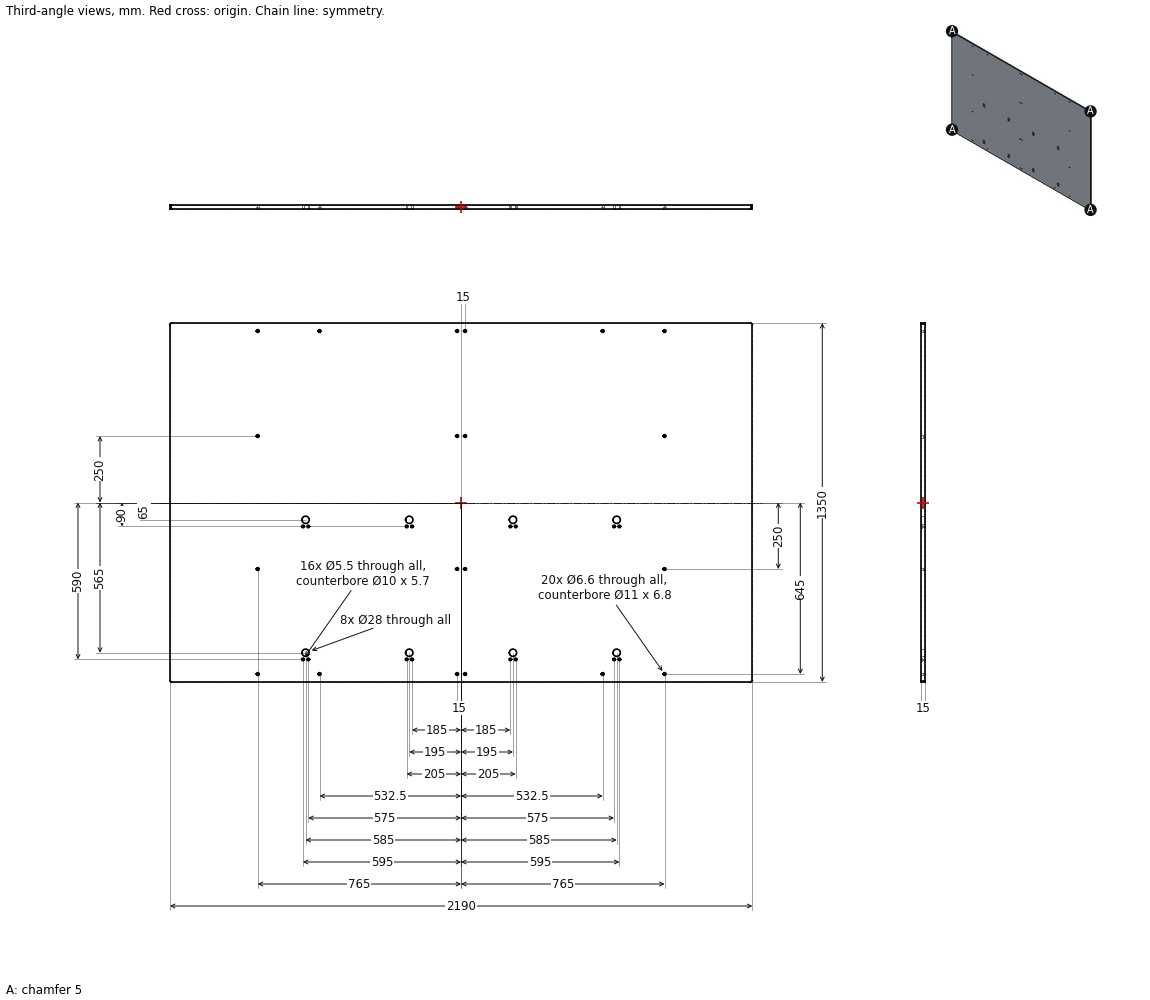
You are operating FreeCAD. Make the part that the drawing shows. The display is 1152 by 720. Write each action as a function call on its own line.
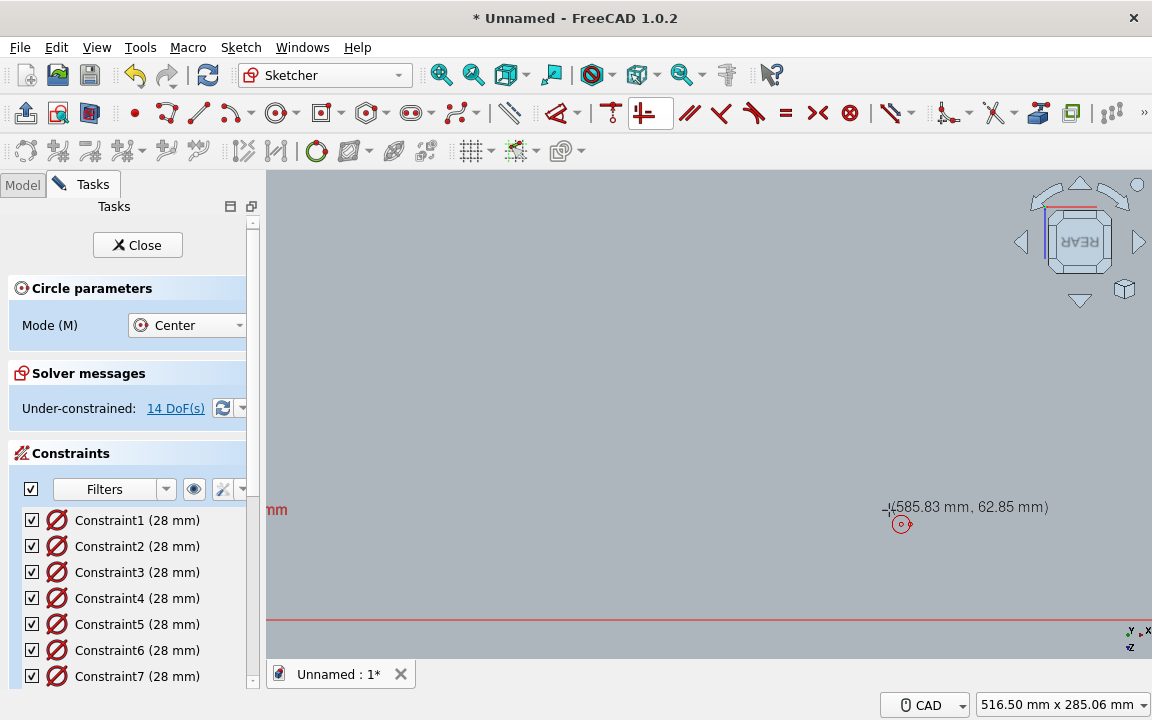
scroll(889, 510, down, 7)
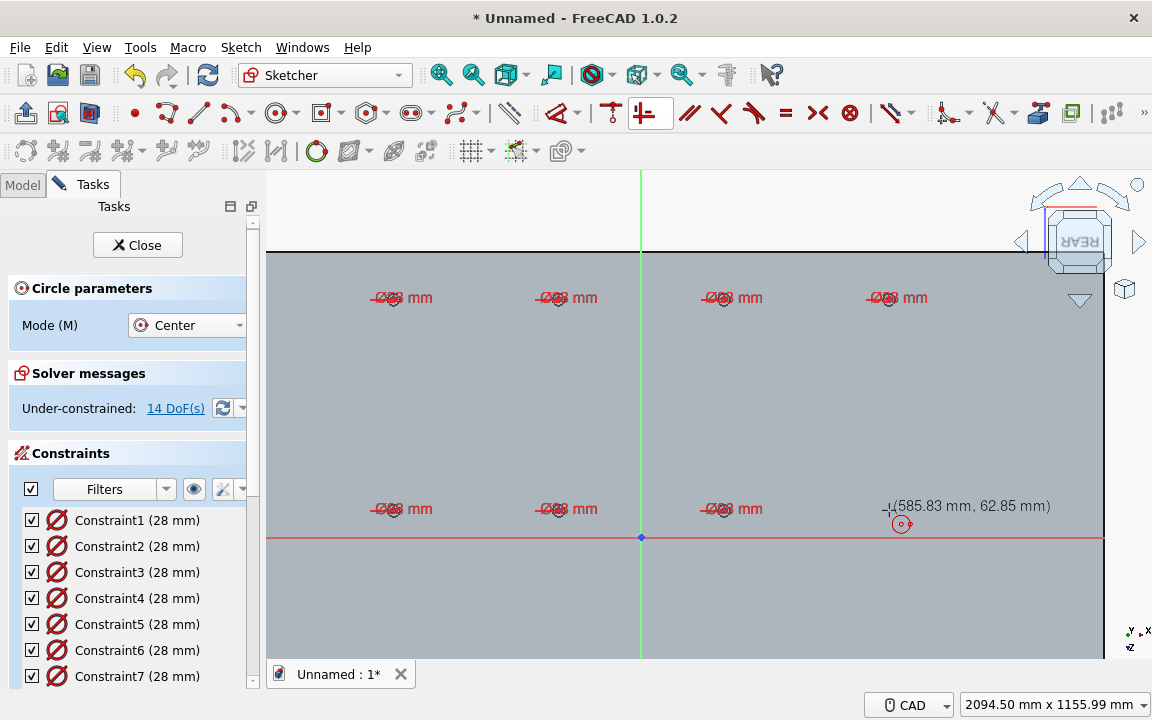
click(889, 510)
move(893, 506)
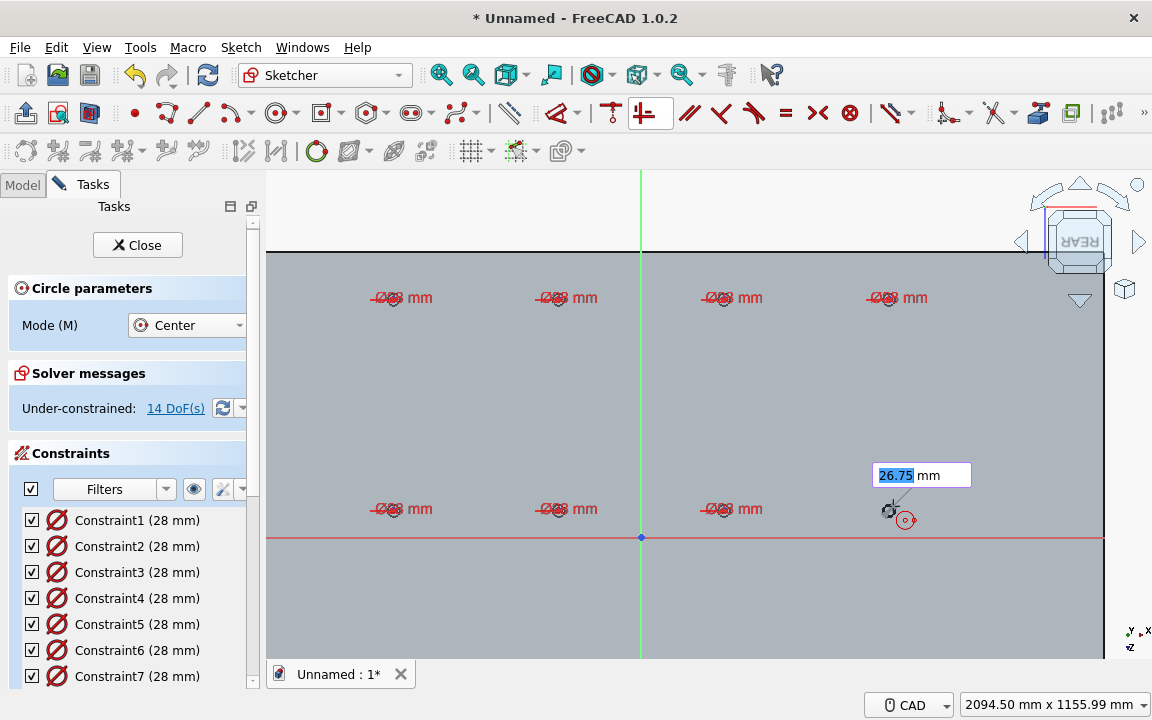
text(28)
key(Return)
key(Escape)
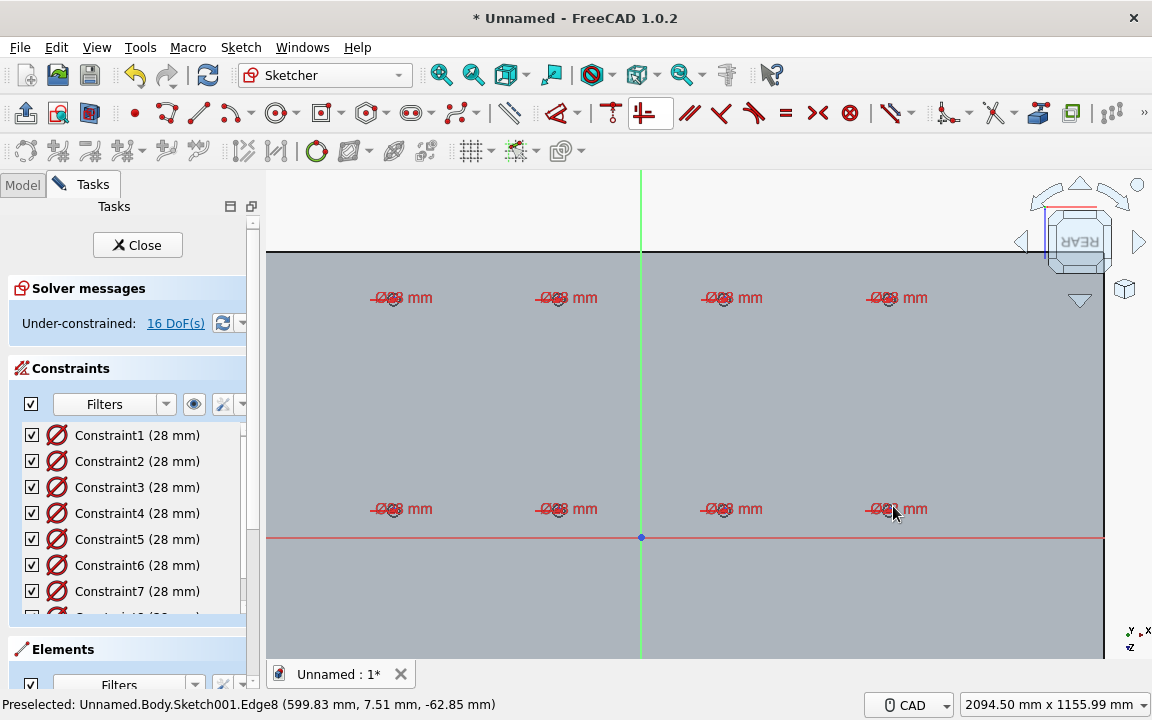
click(394, 300)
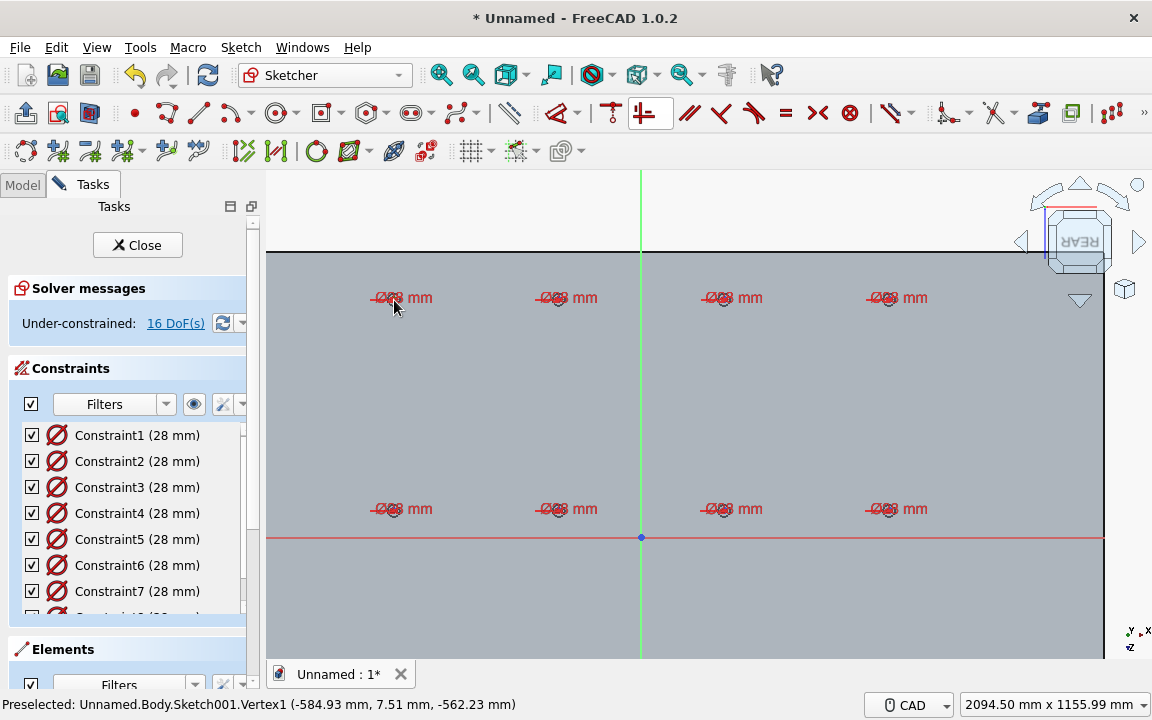
click(559, 300)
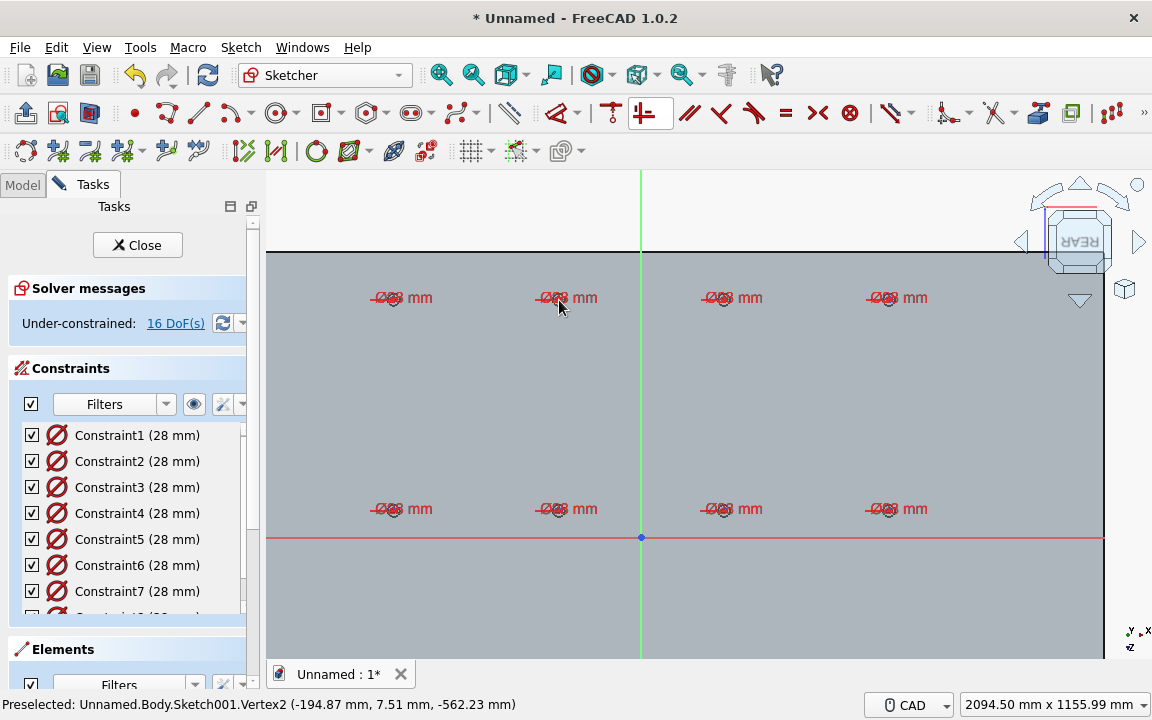
key(h)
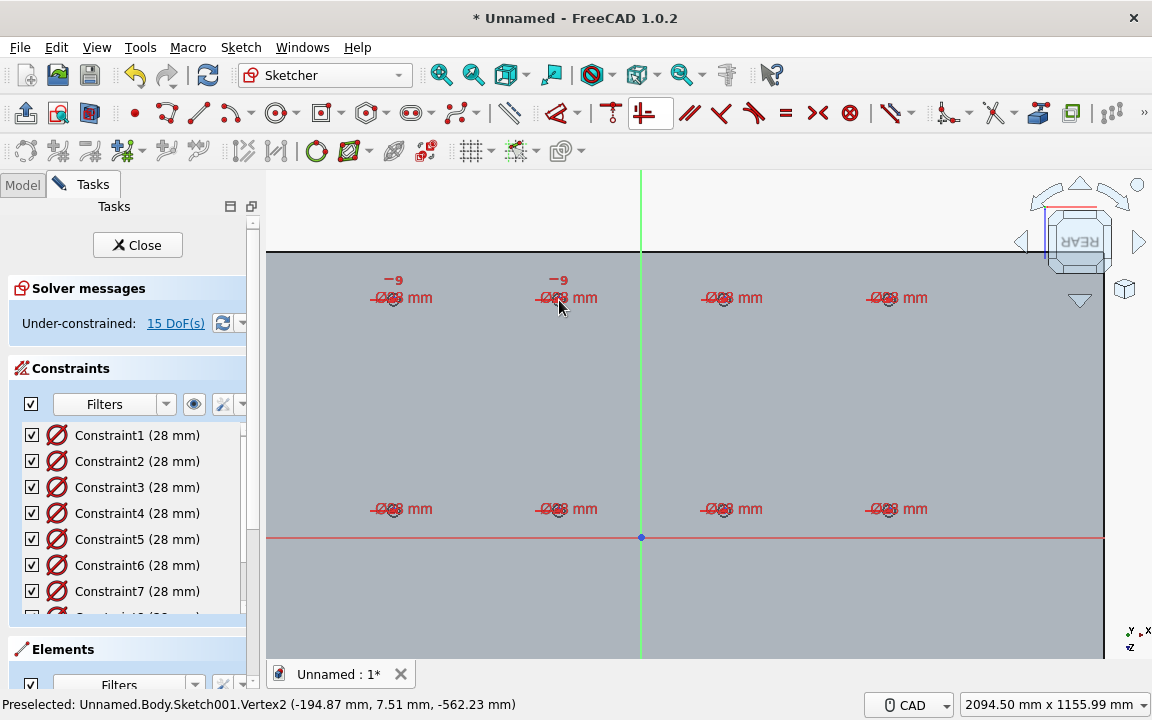
click(559, 300)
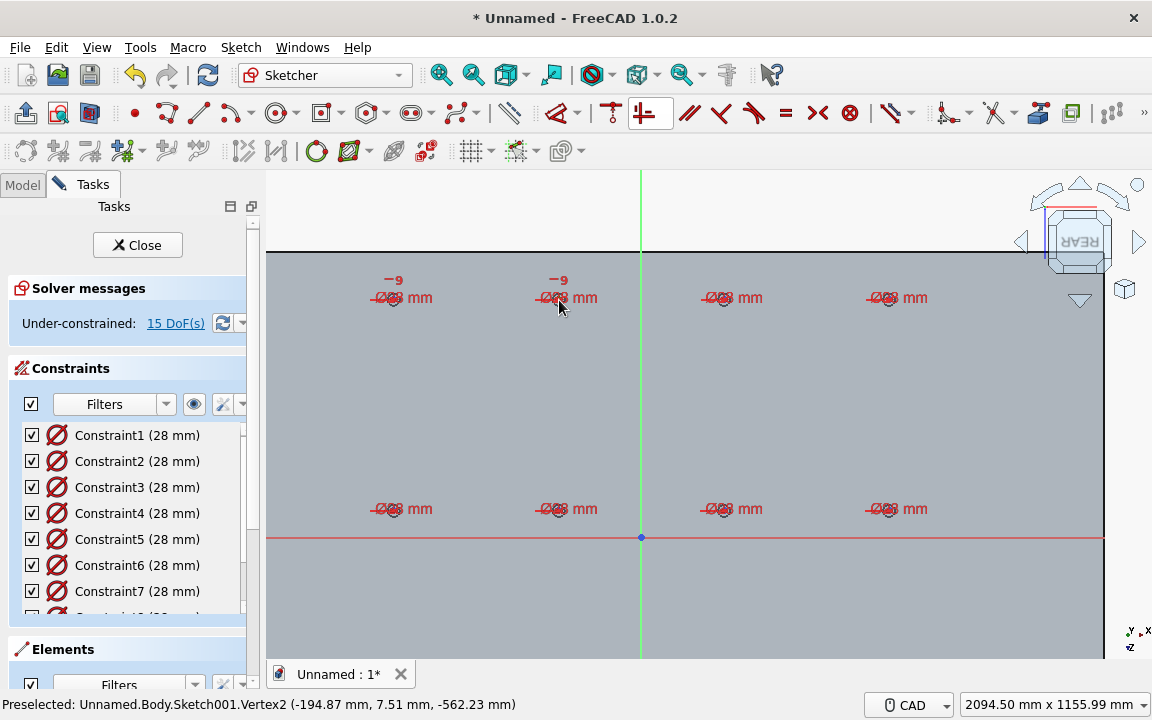
click(724, 300)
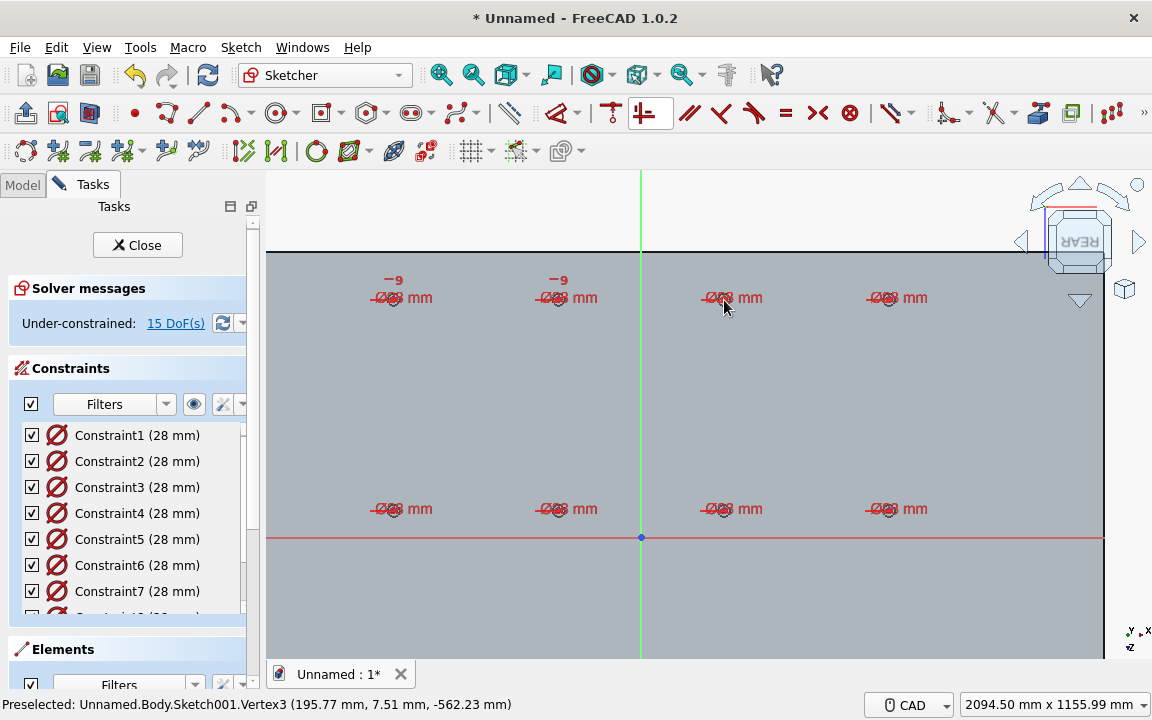
click(668, 114)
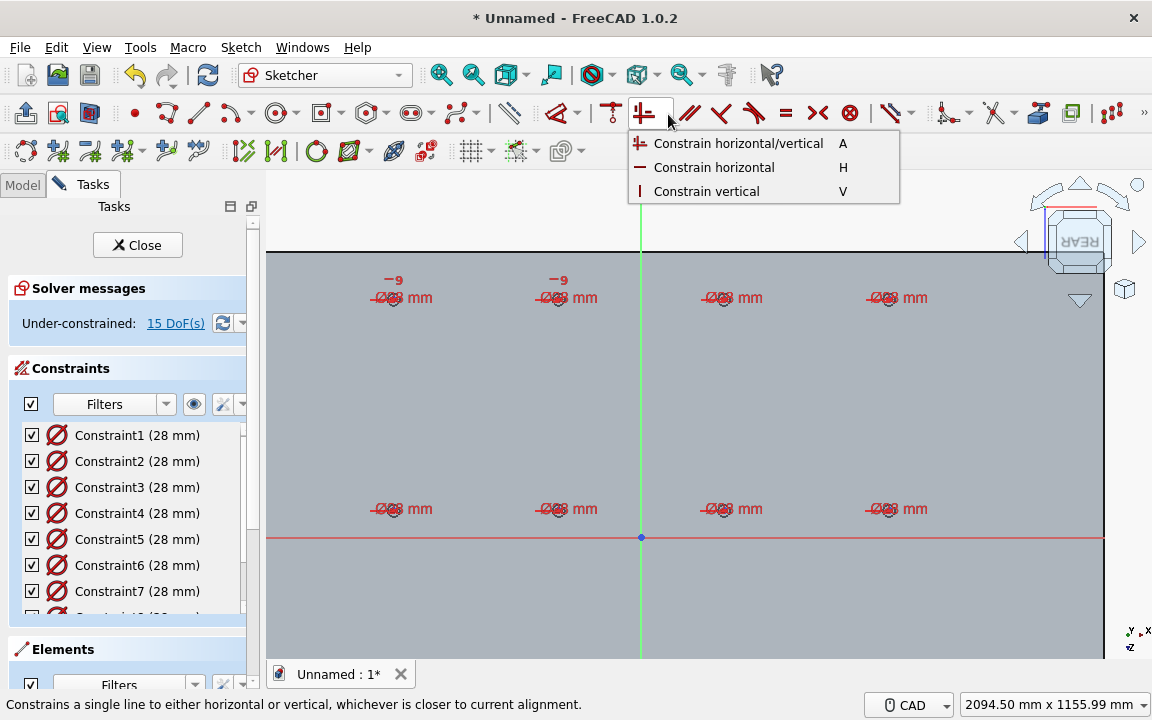
click(764, 167)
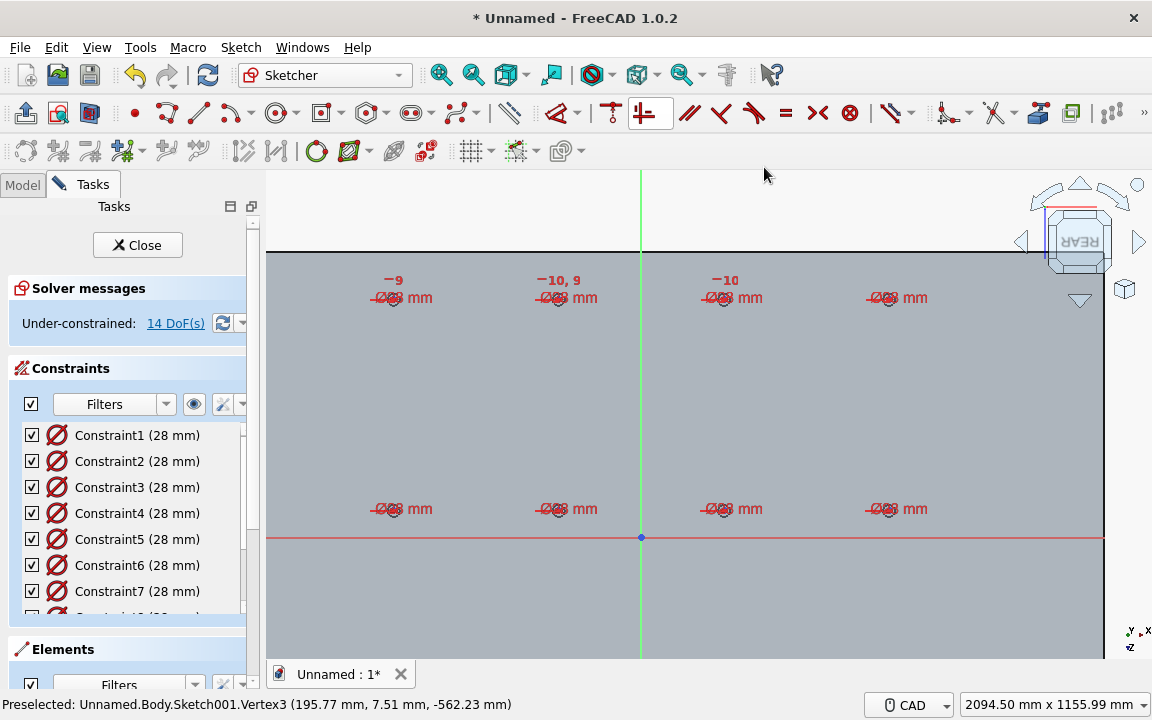
click(724, 300)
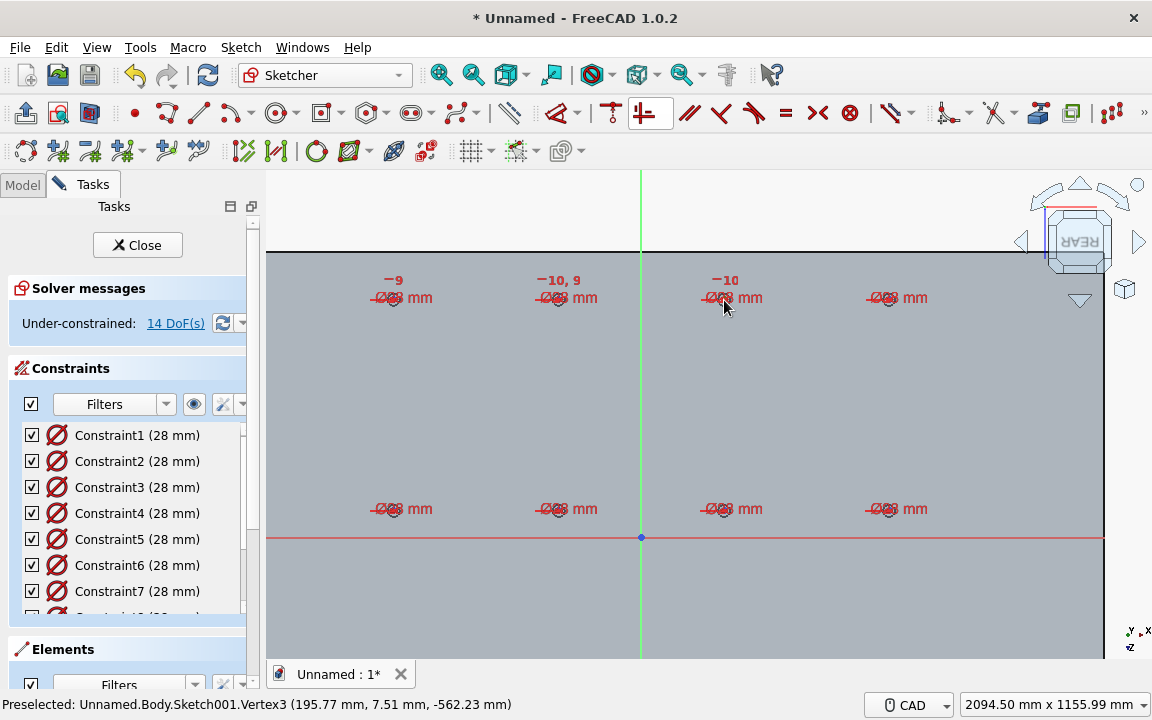
click(889, 300)